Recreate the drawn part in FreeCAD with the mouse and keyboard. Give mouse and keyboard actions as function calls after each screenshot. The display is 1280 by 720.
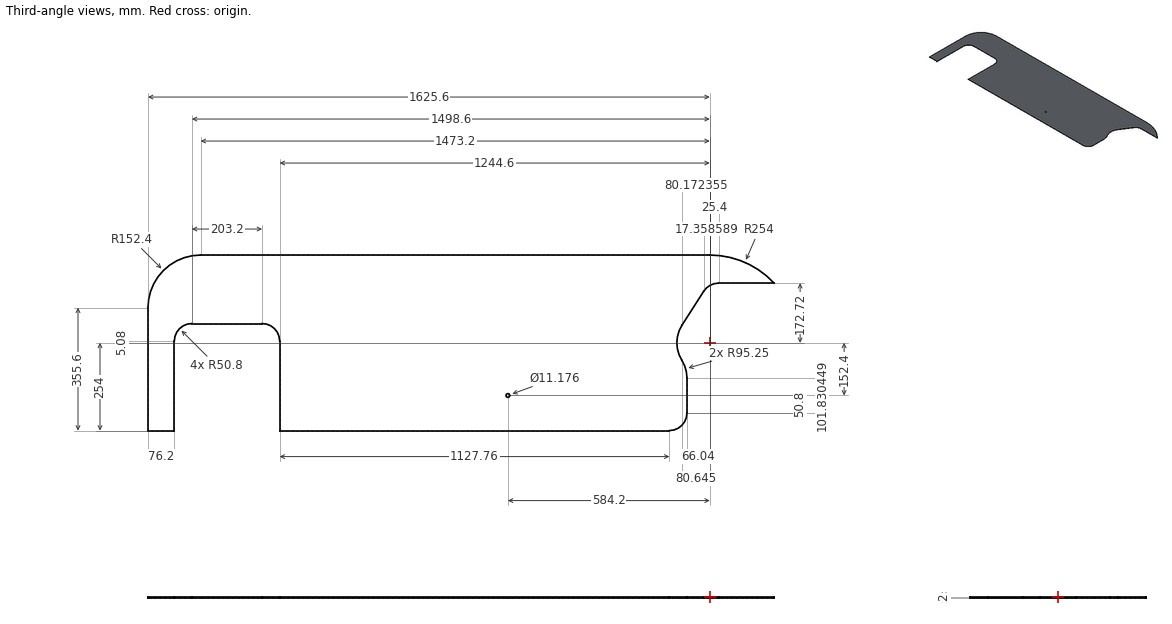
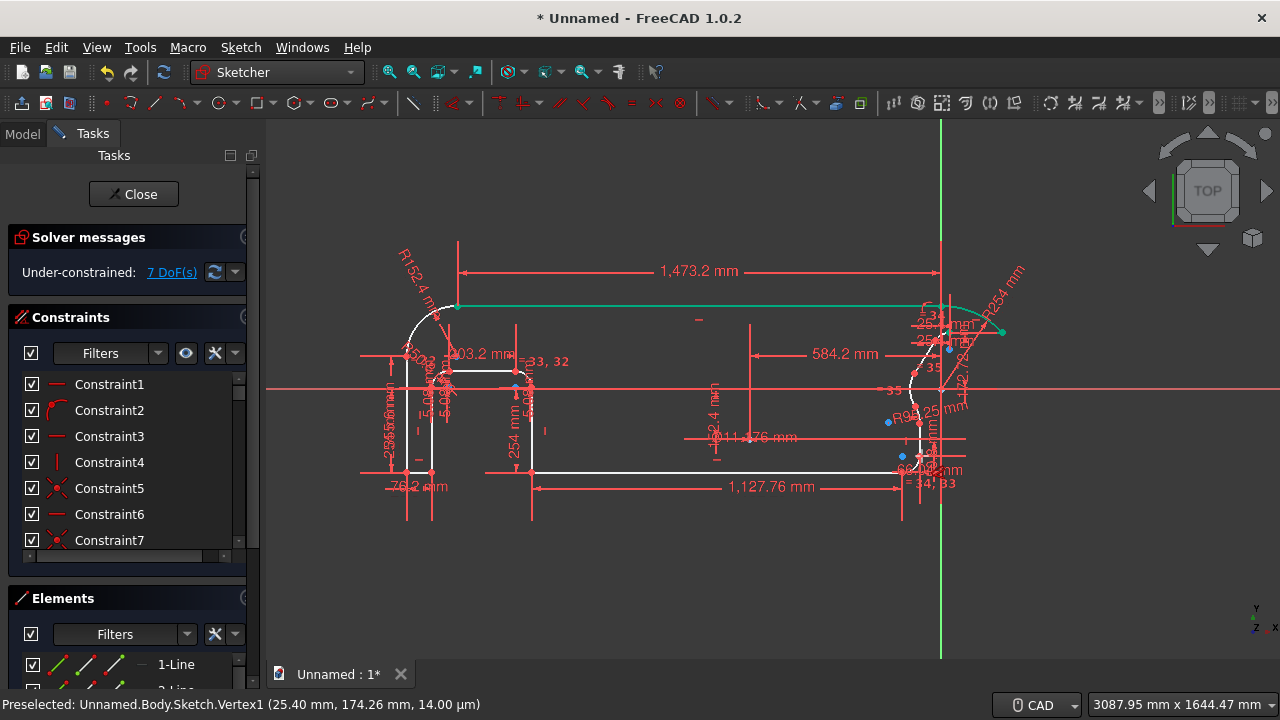
click(407, 356)
click(674, 322)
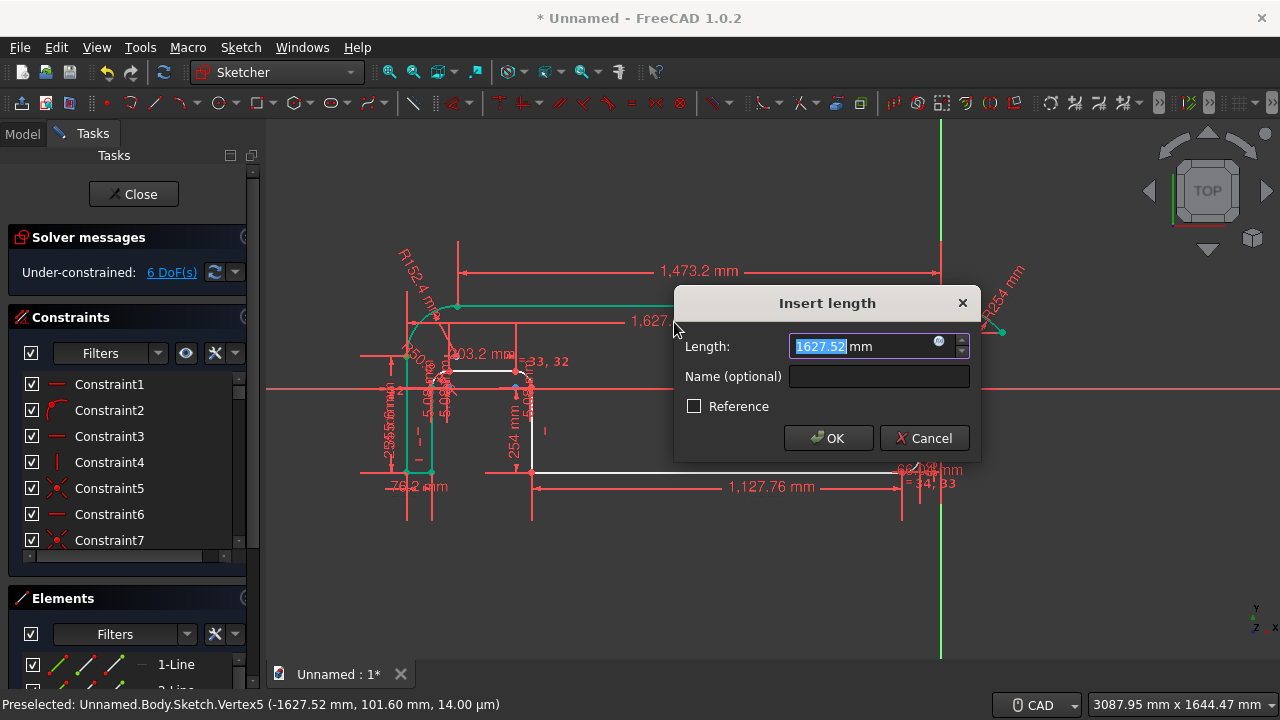
text(1625.6)
key(Return)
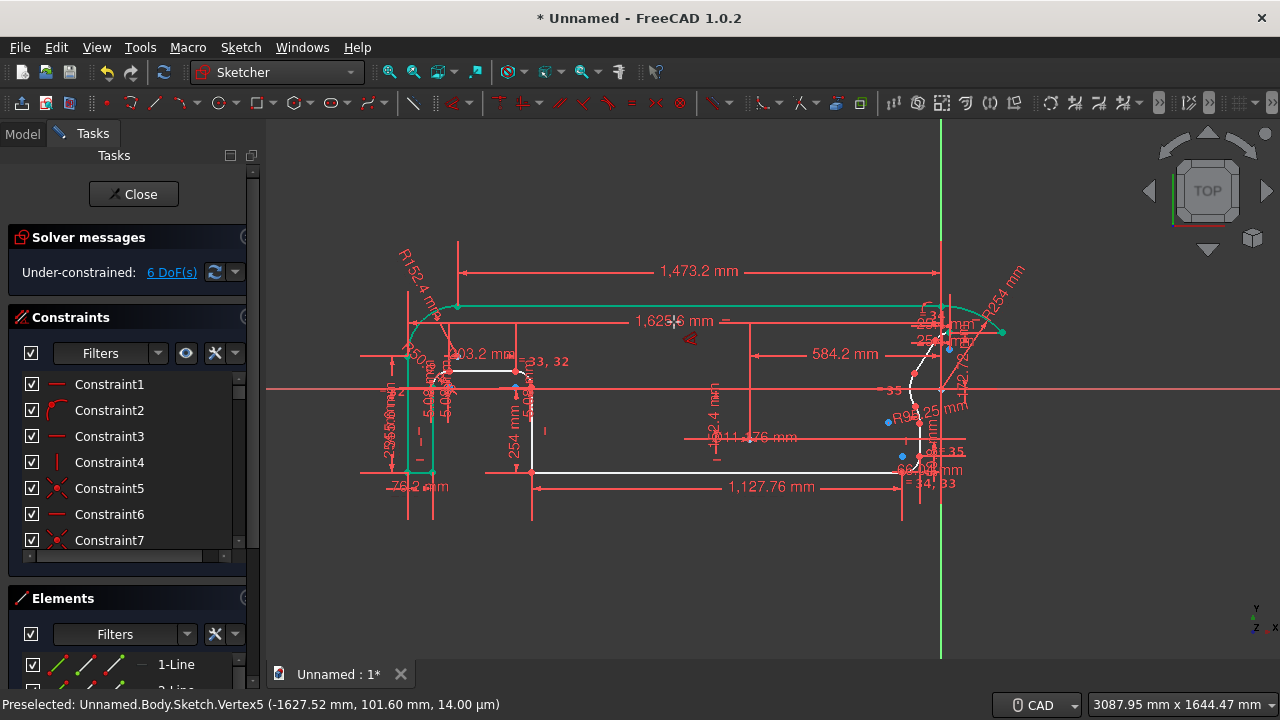
click(449, 371)
click(582, 337)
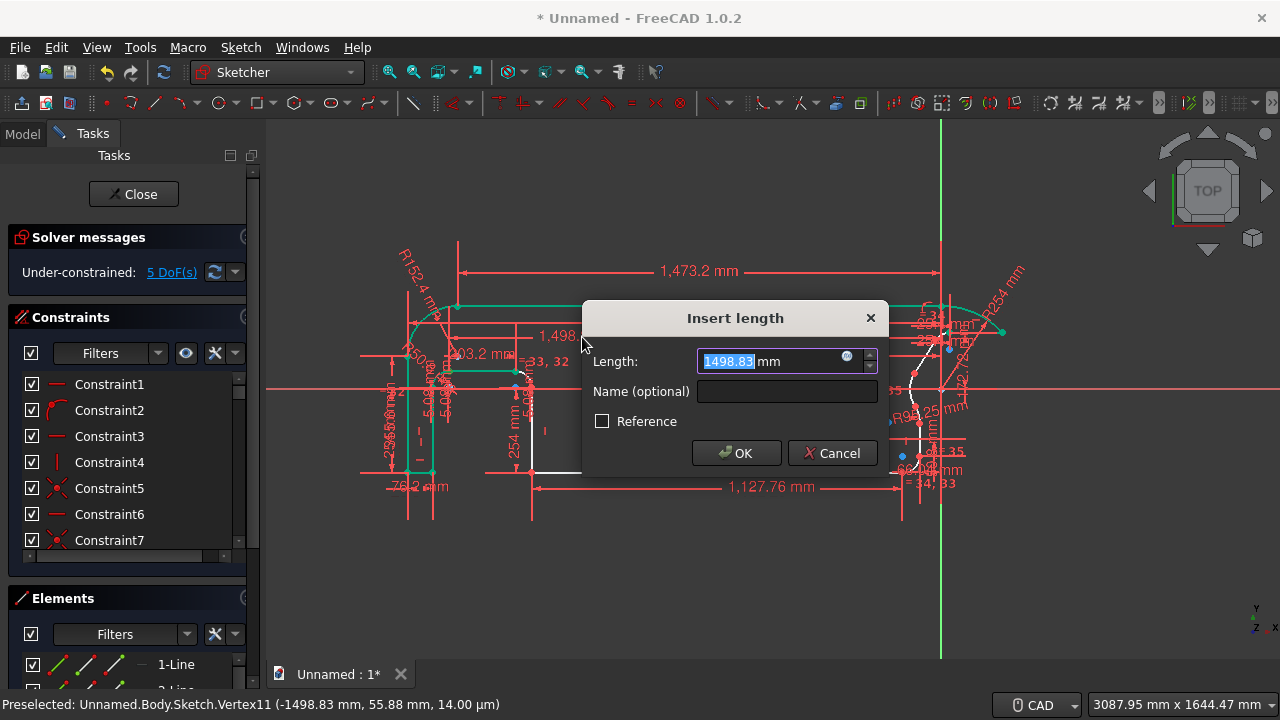
text(1498.6)
key(Return)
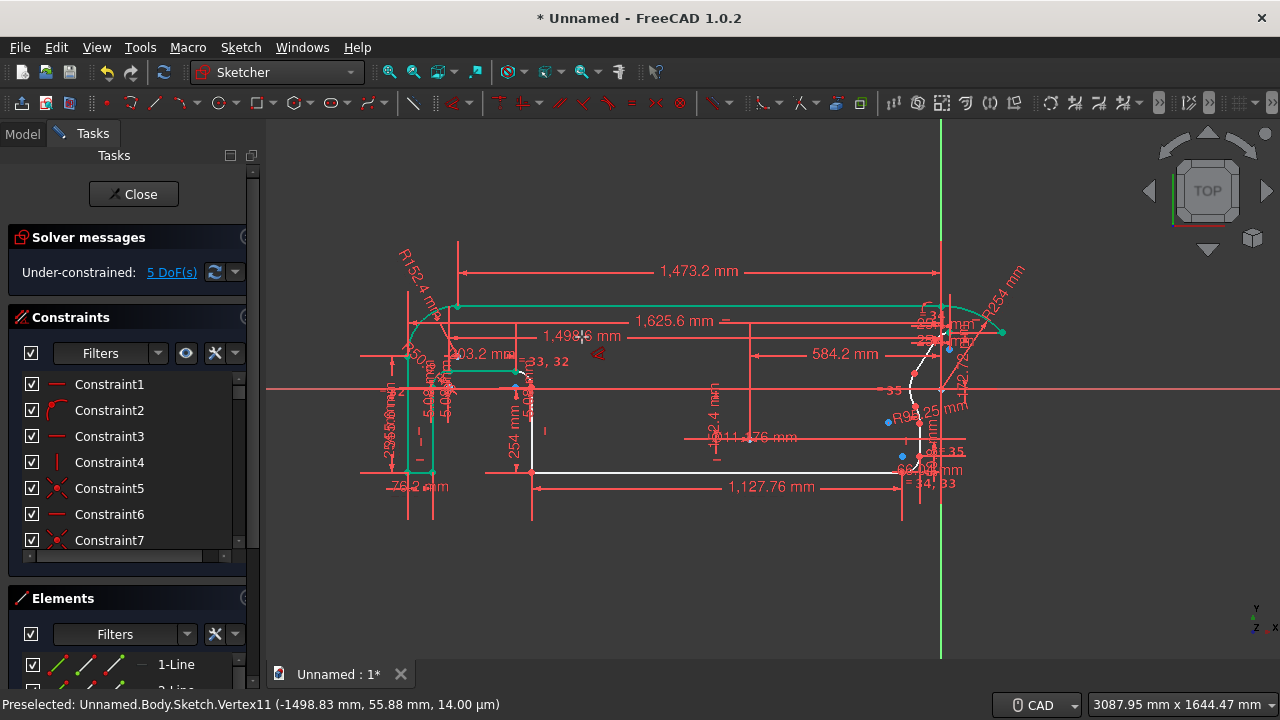
click(532, 388)
click(737, 354)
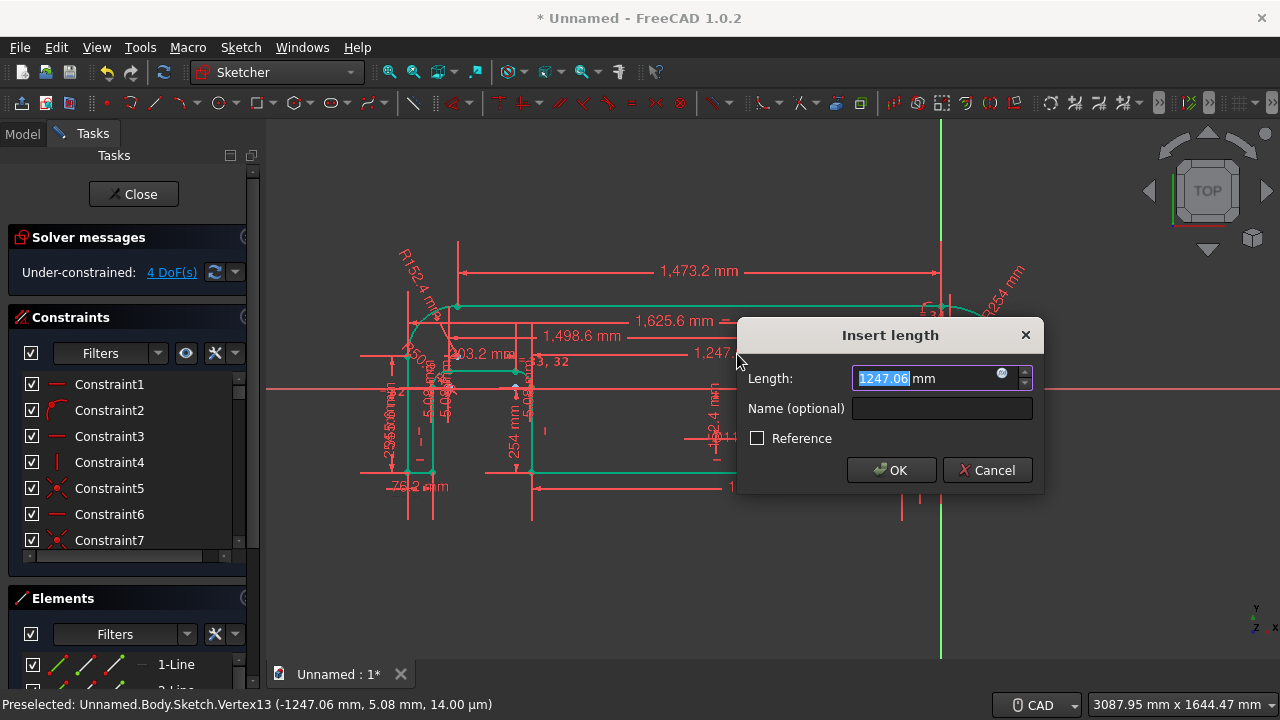
text(1244.6)
key(Return)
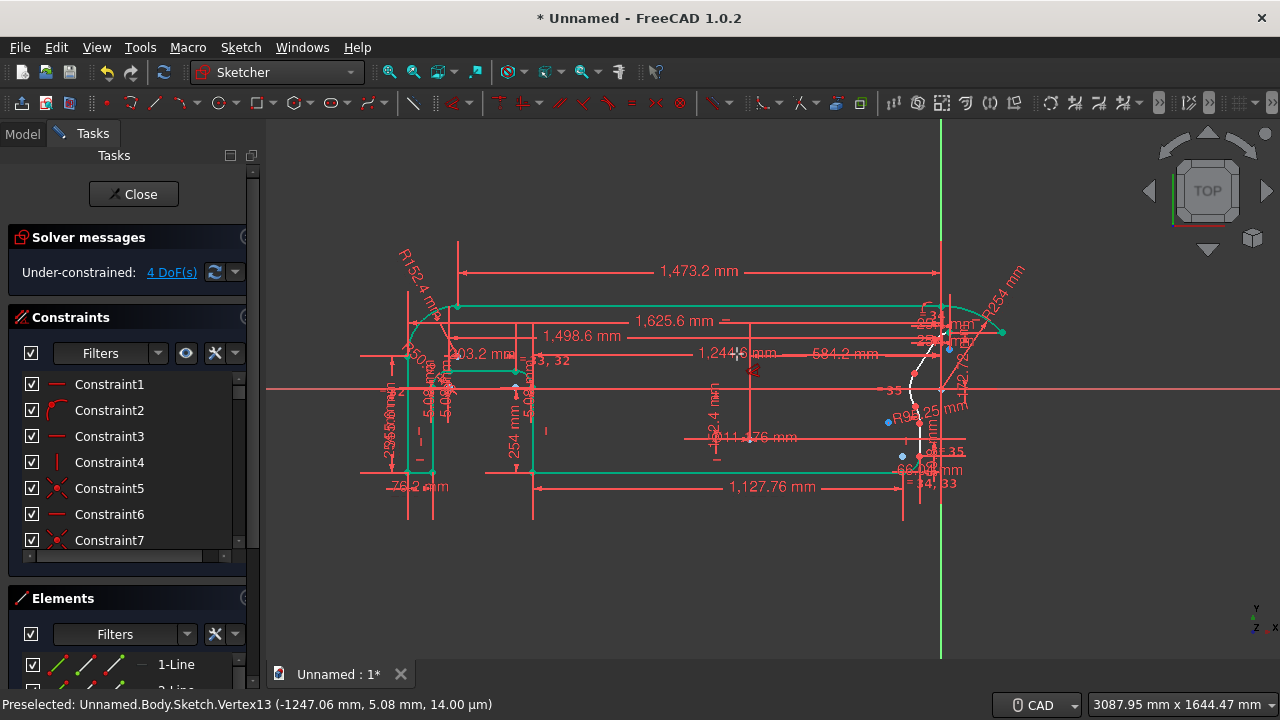
scroll(915, 406, up, 3)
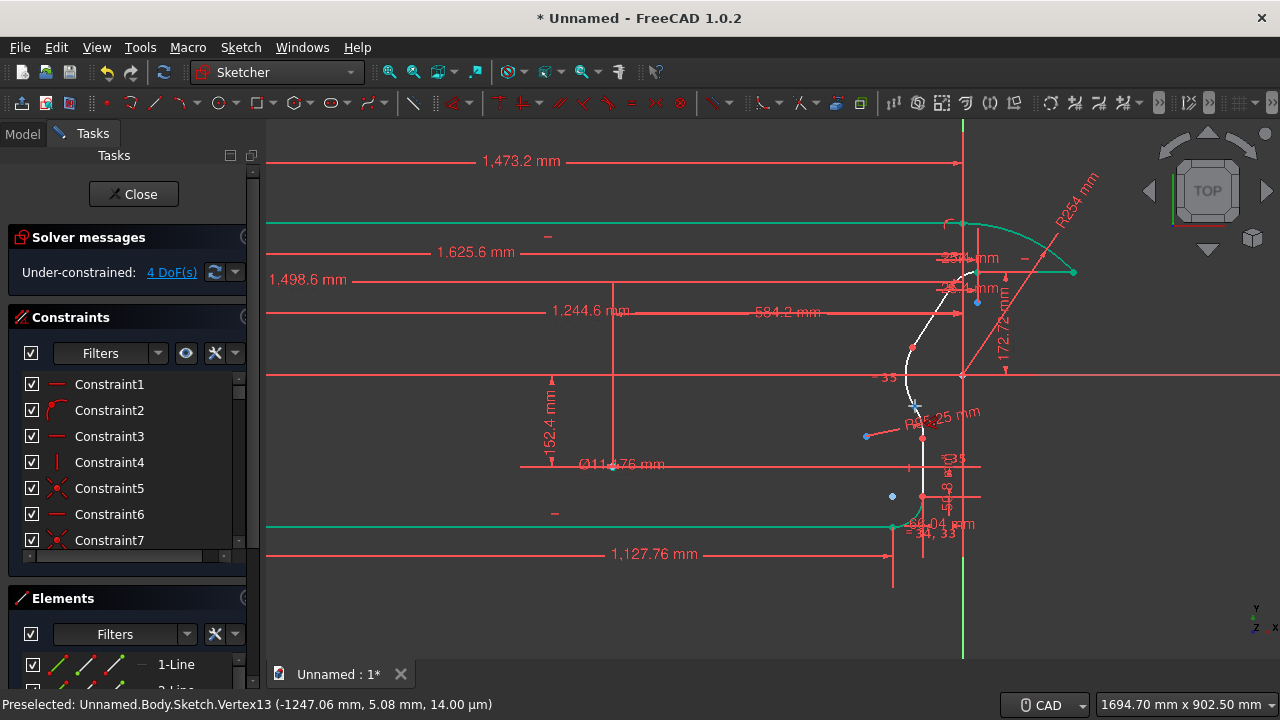
click(915, 406)
click(939, 560)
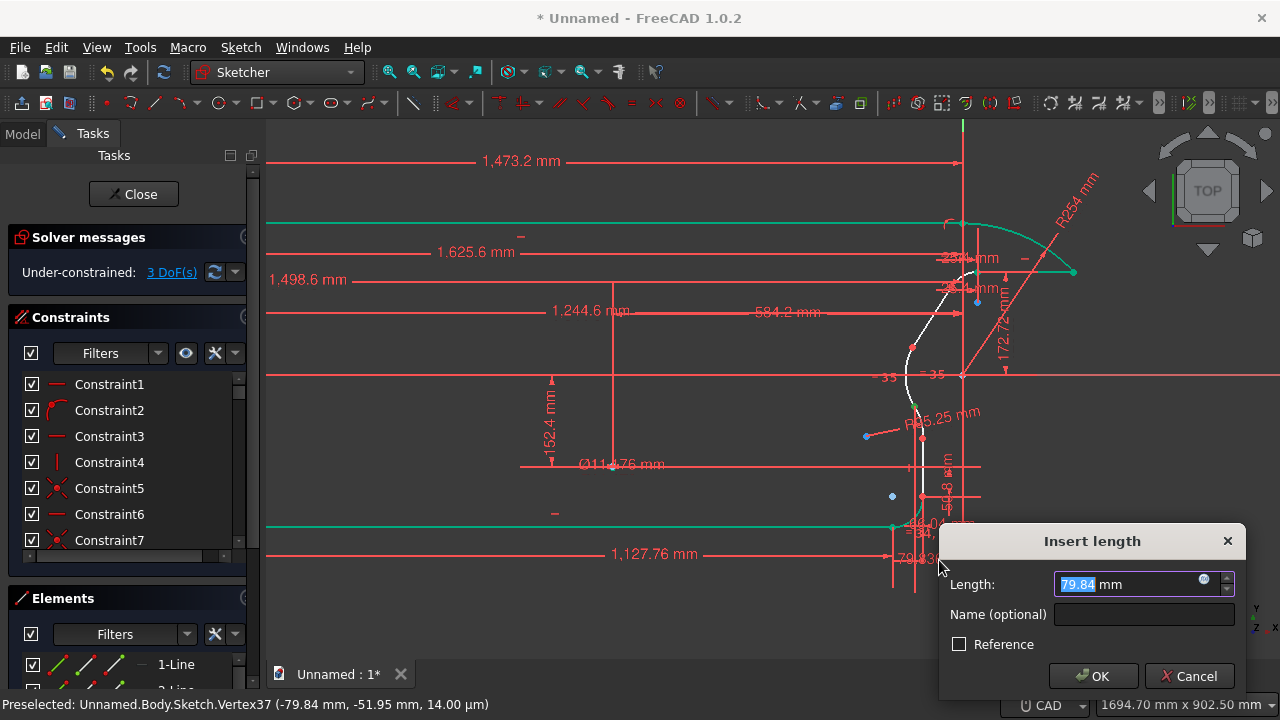
text(80.645)
key(Return)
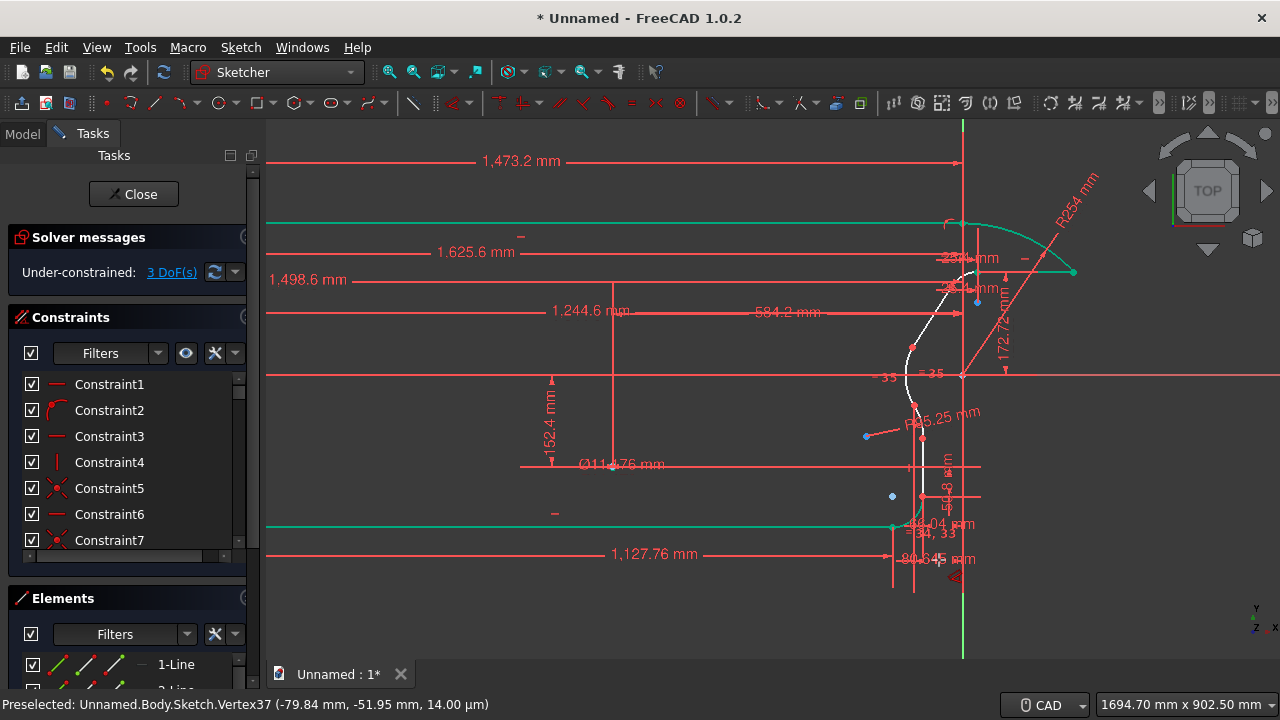
click(923, 479)
click(889, 454)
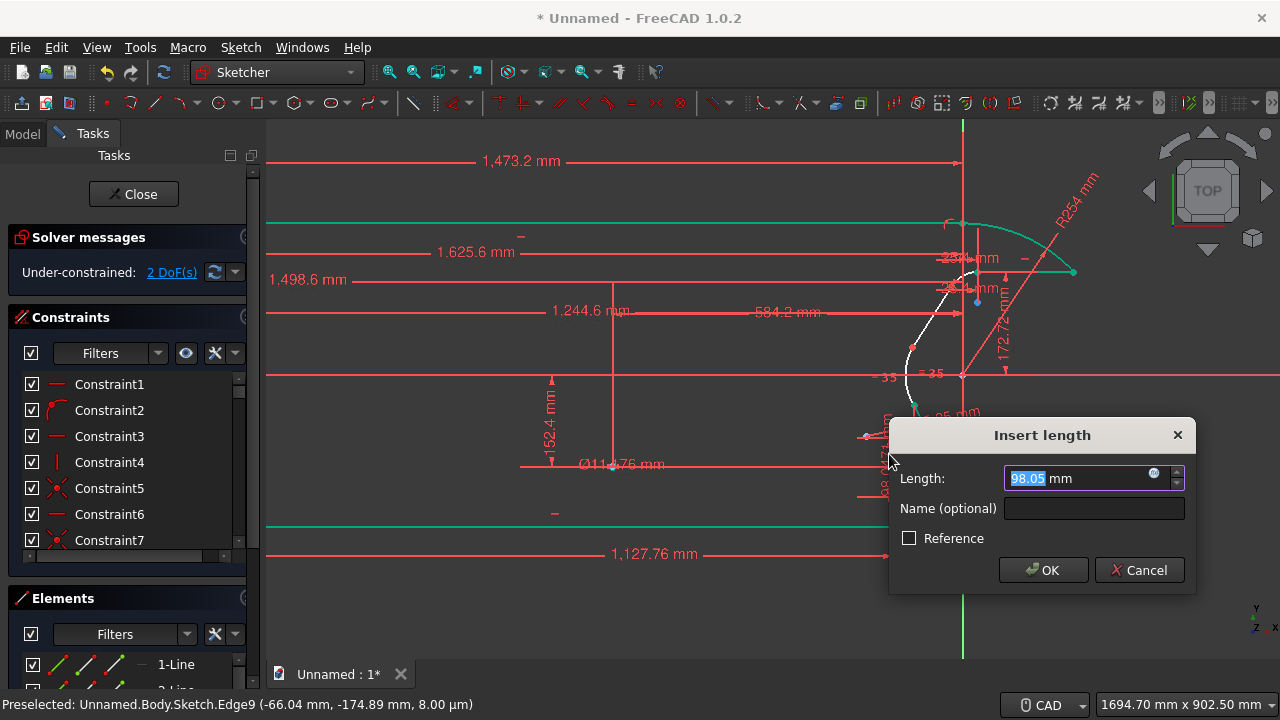
text(101.830449)
key(Return)